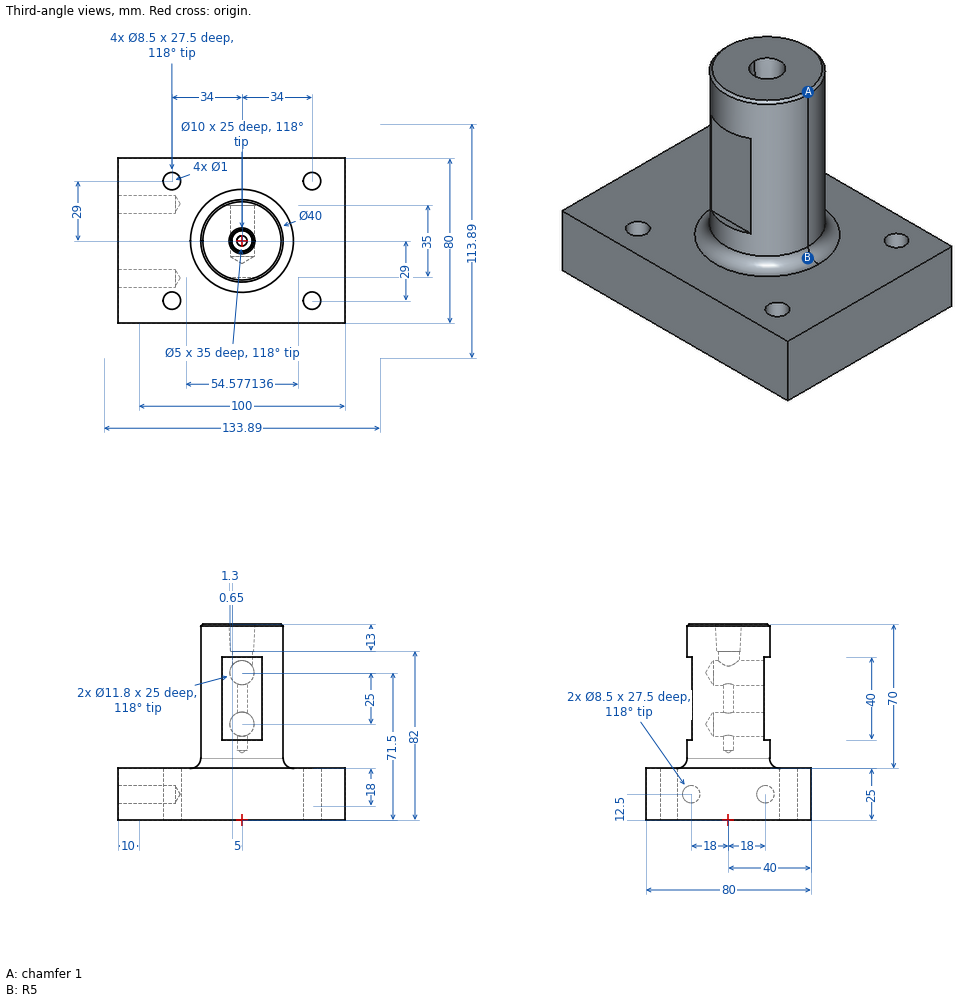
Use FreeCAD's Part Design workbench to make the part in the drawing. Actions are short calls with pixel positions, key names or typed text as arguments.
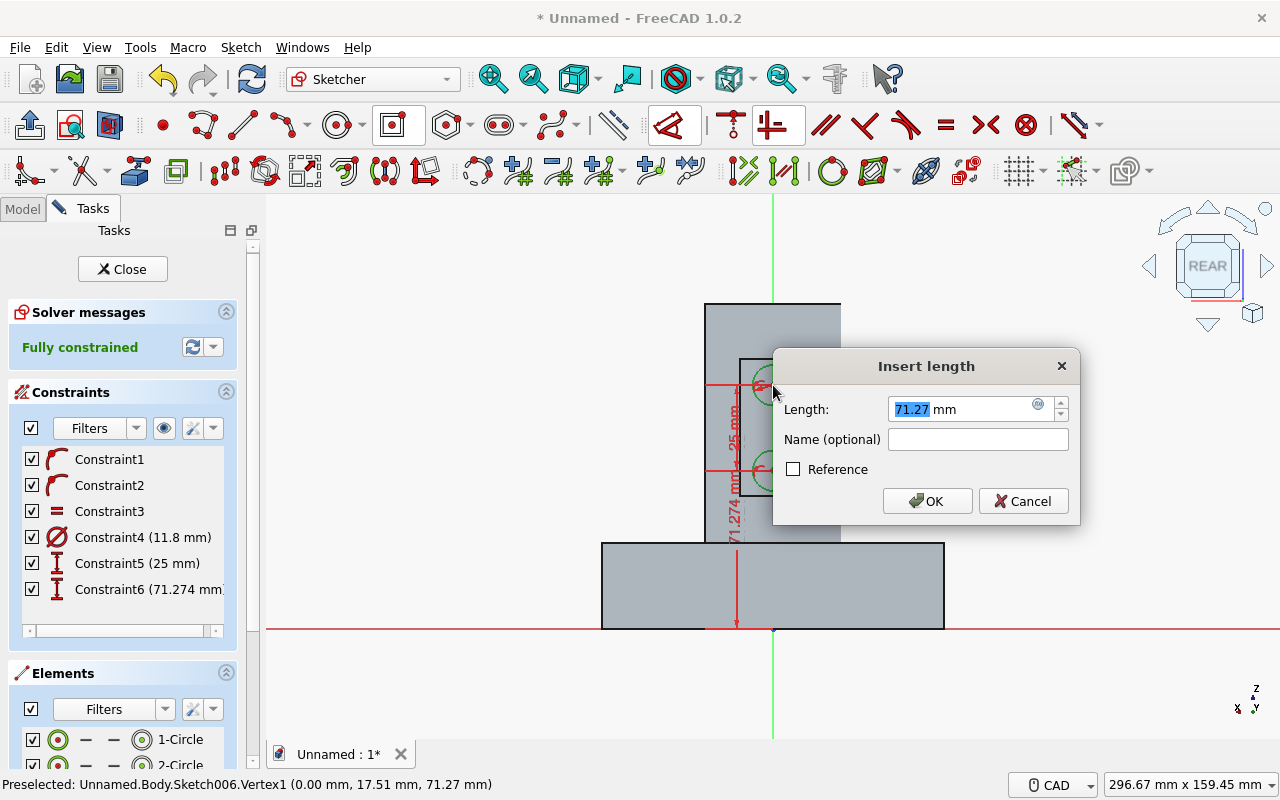
text(71.5)
key(Return)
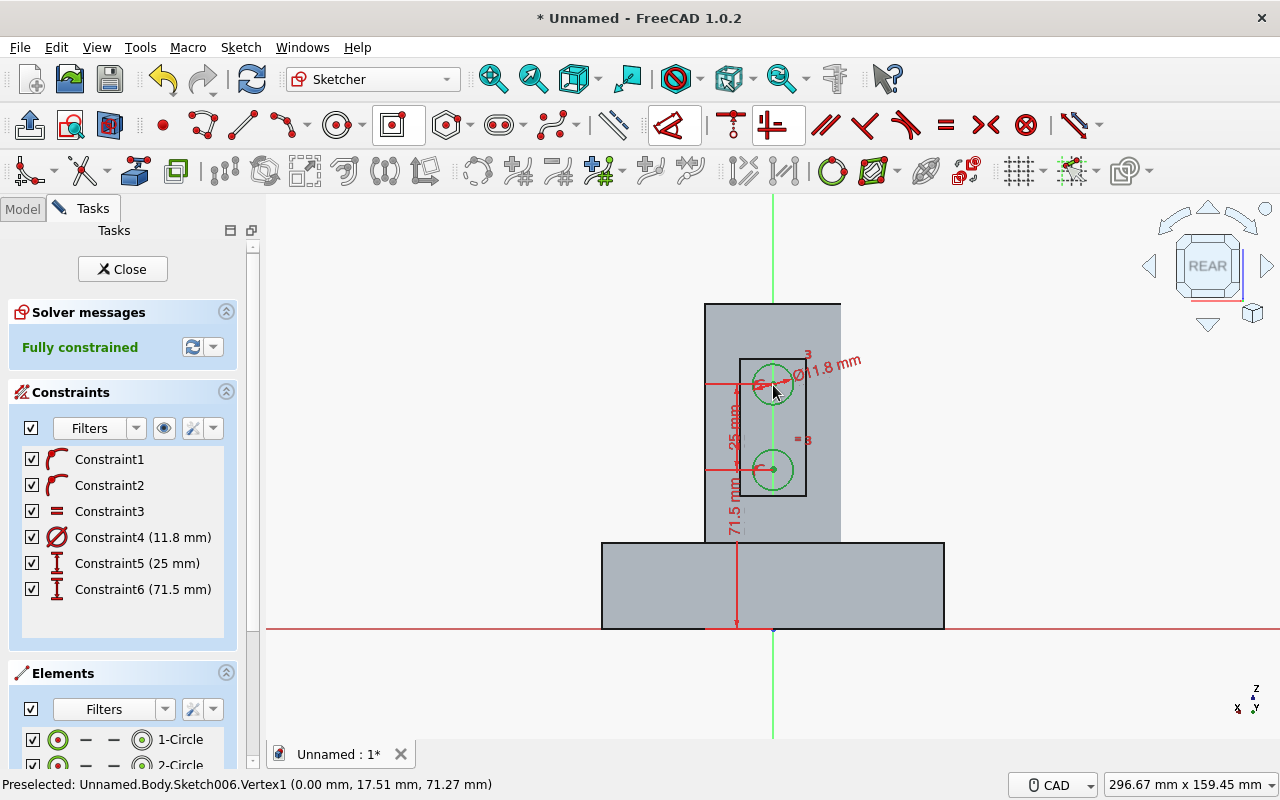
click(123, 269)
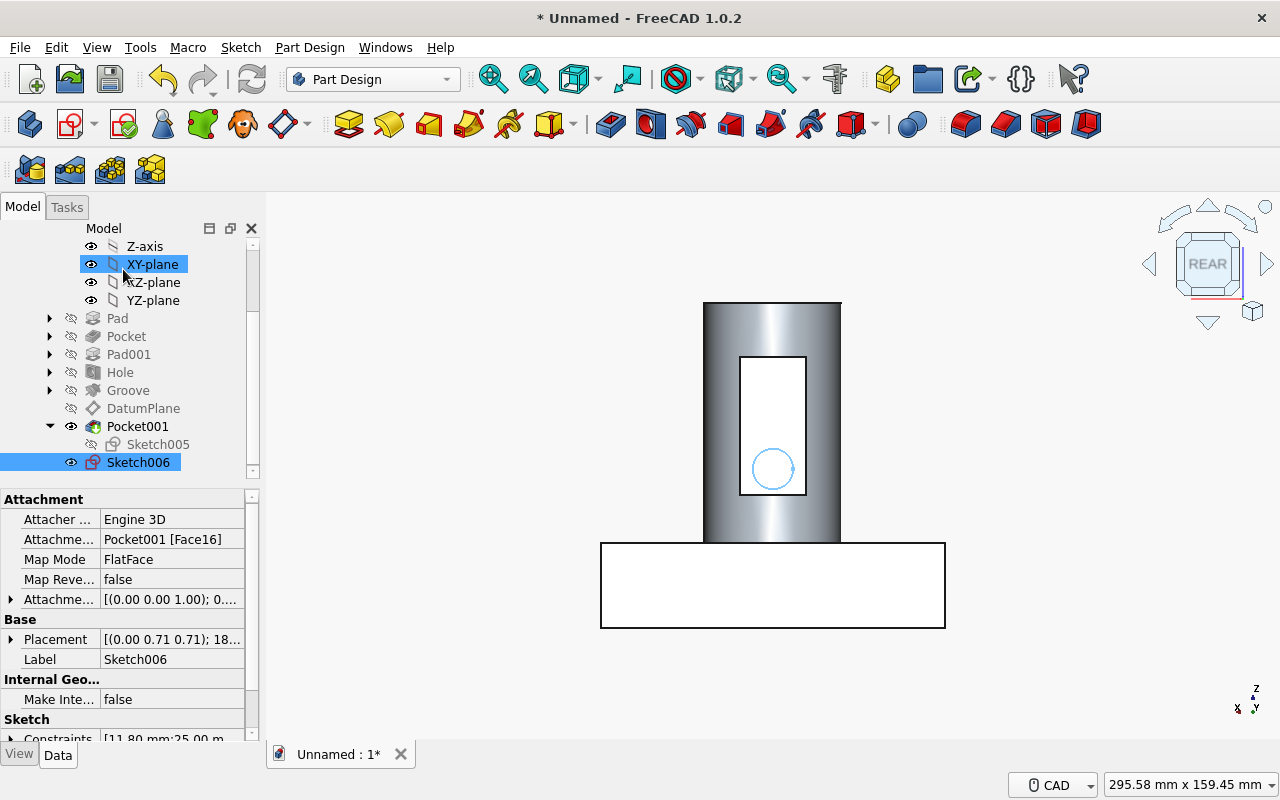
click(652, 124)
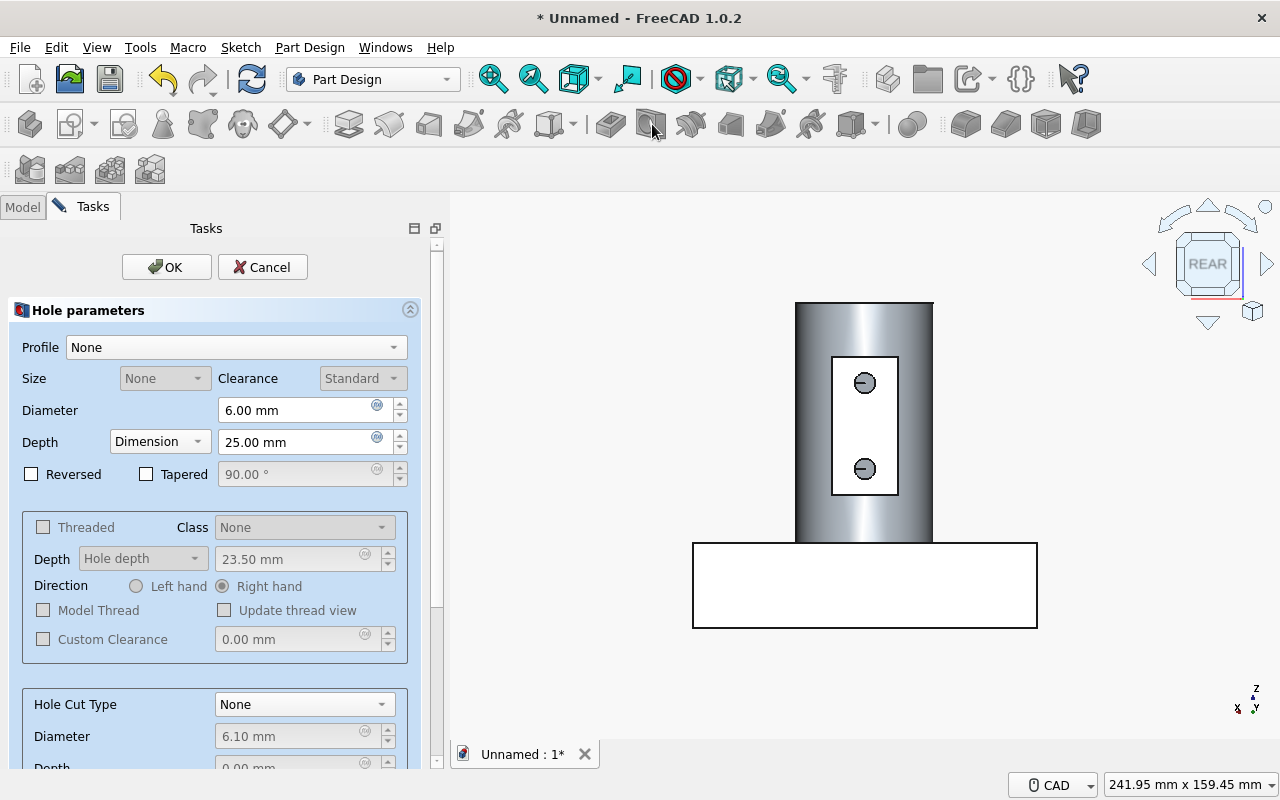
triple_click(305, 410)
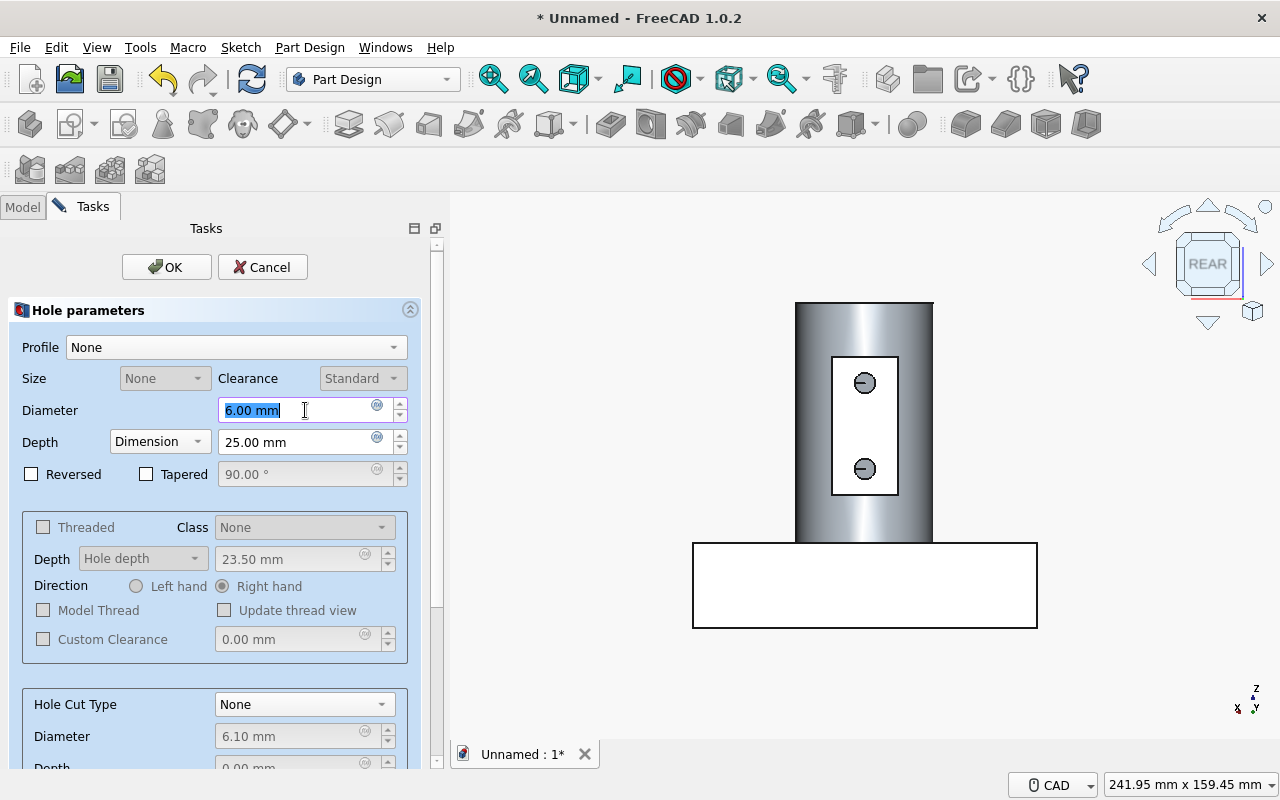
text(11.8)
key(Tab)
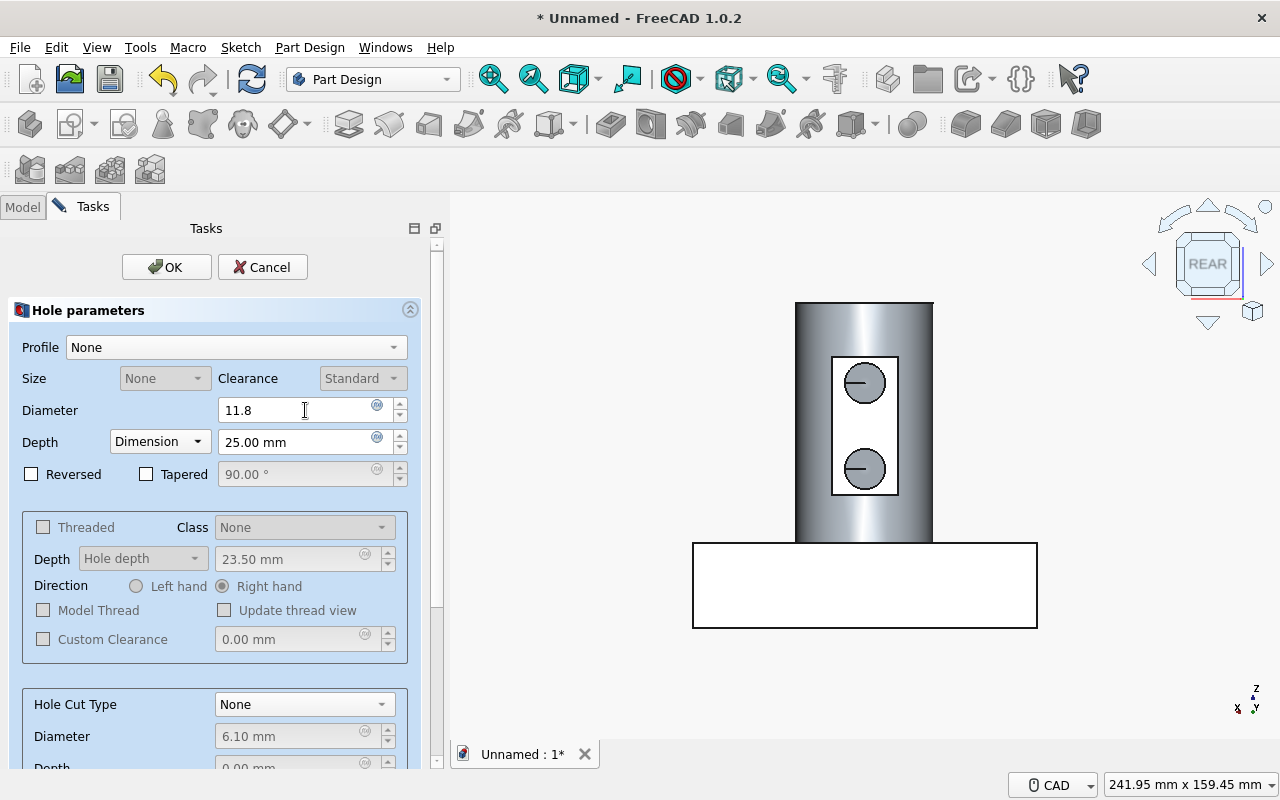
triple_click(305, 442)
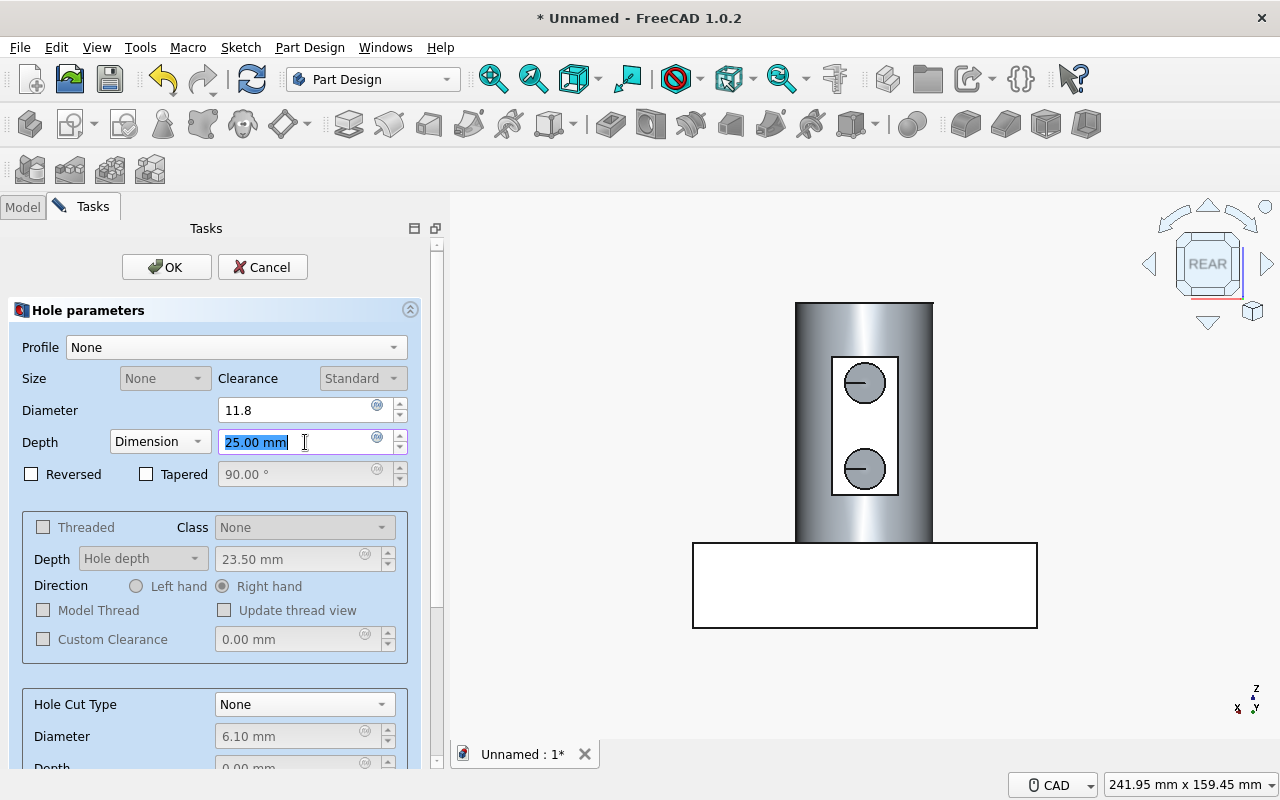
text(25)
key(Tab)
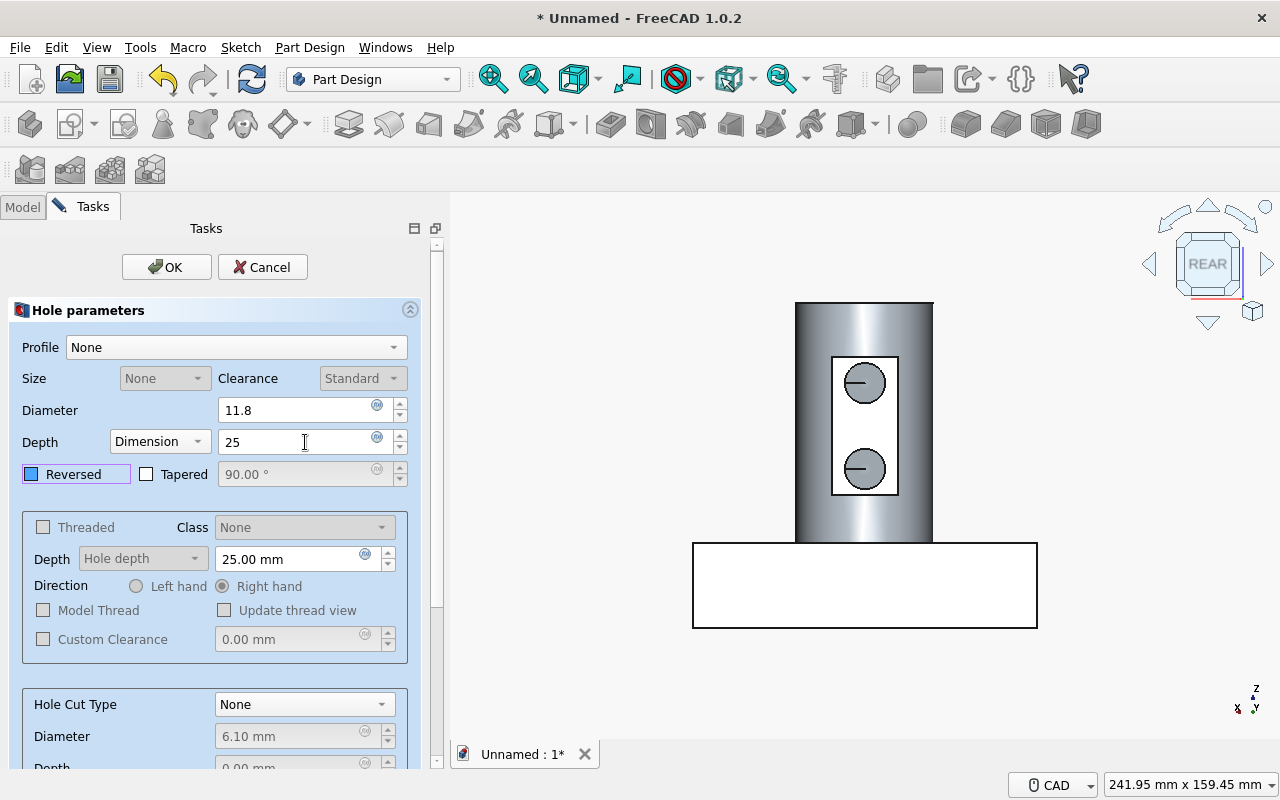
click(167, 267)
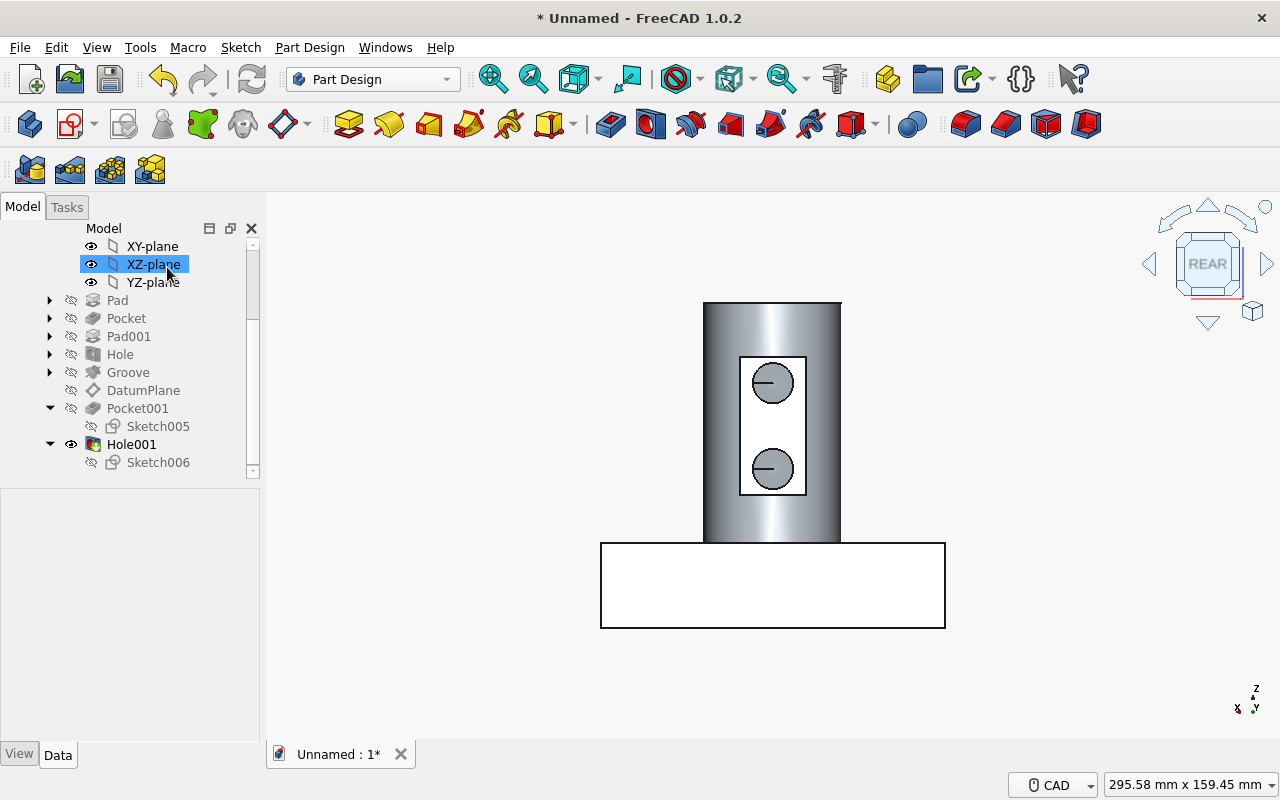
click(829, 302)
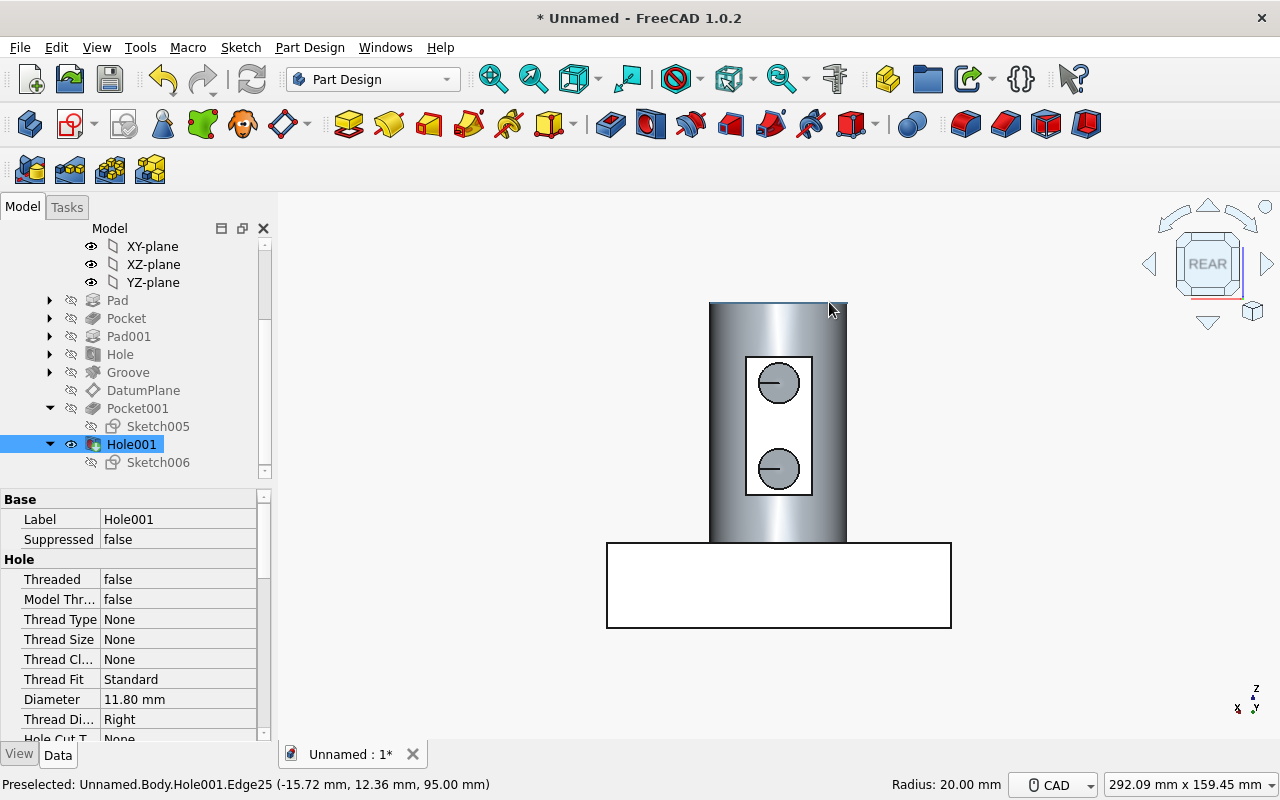
click(1006, 124)